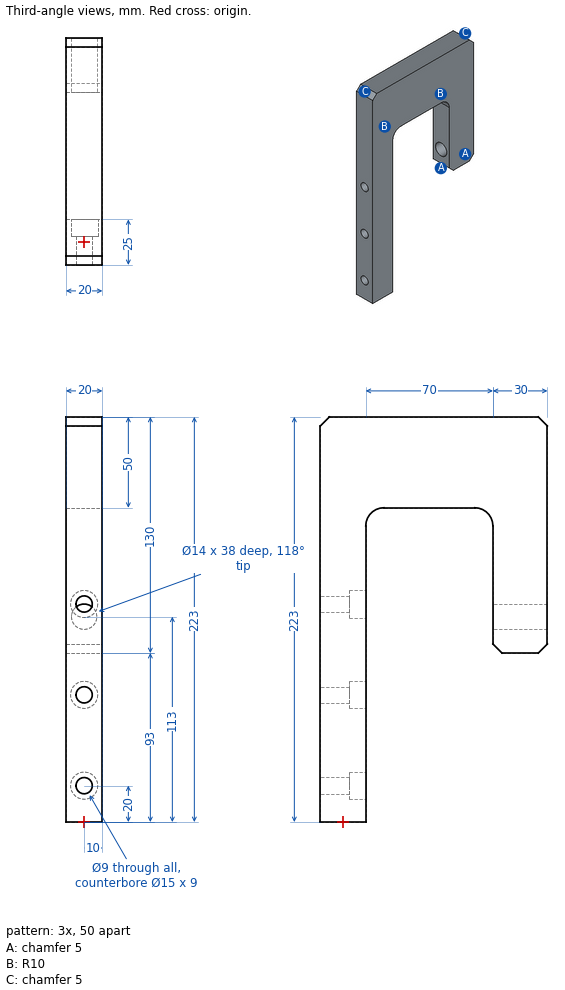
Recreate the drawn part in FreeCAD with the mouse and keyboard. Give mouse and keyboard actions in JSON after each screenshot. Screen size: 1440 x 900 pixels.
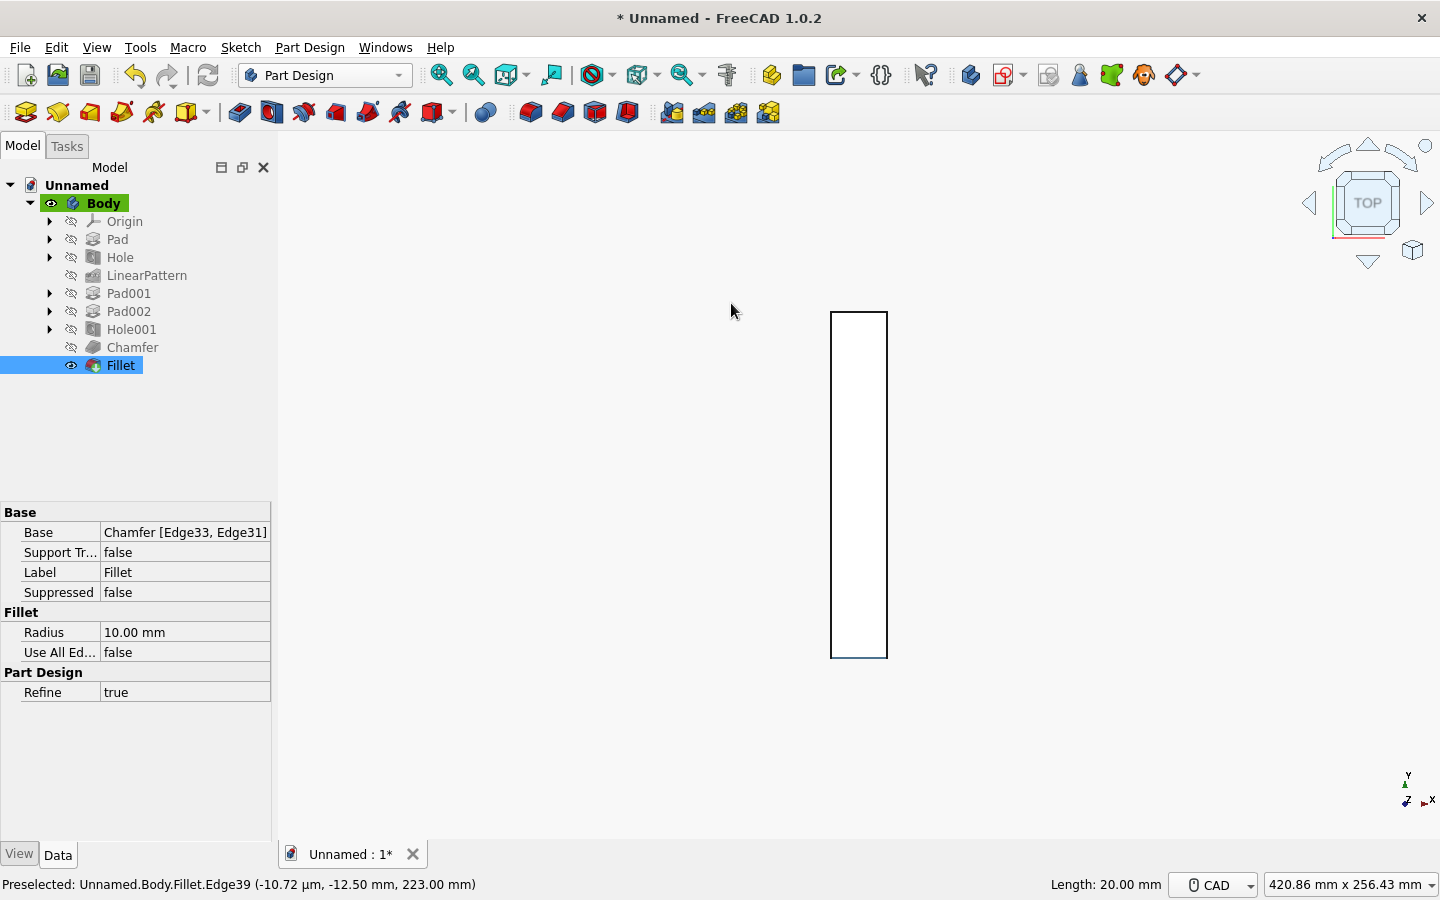
{"action": "left_click", "coordinate": [859, 311], "text": "ctrl"}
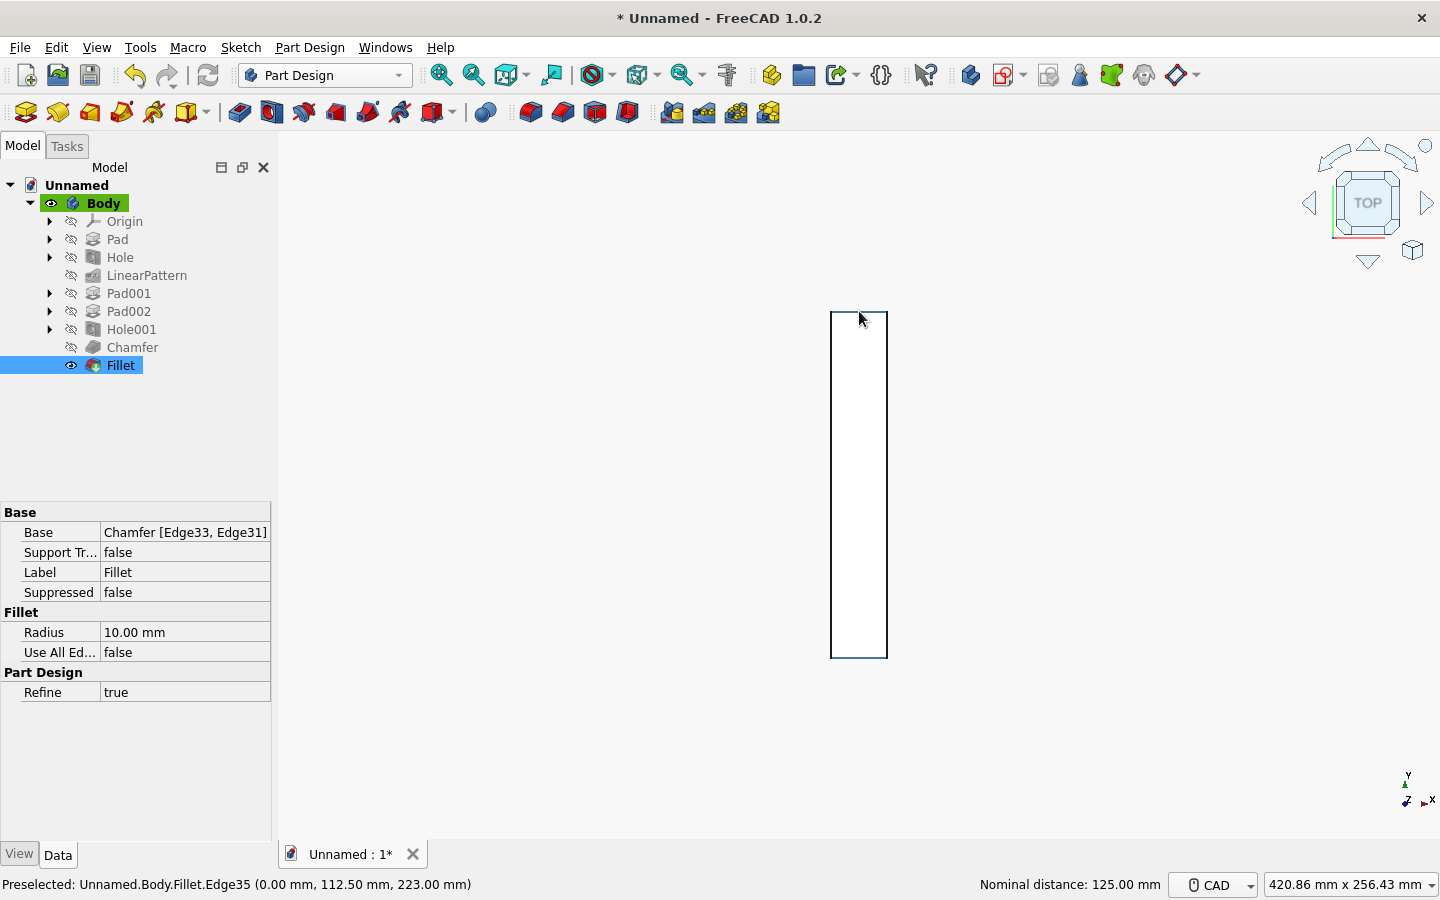
{"action": "left_click", "coordinate": [564, 112]}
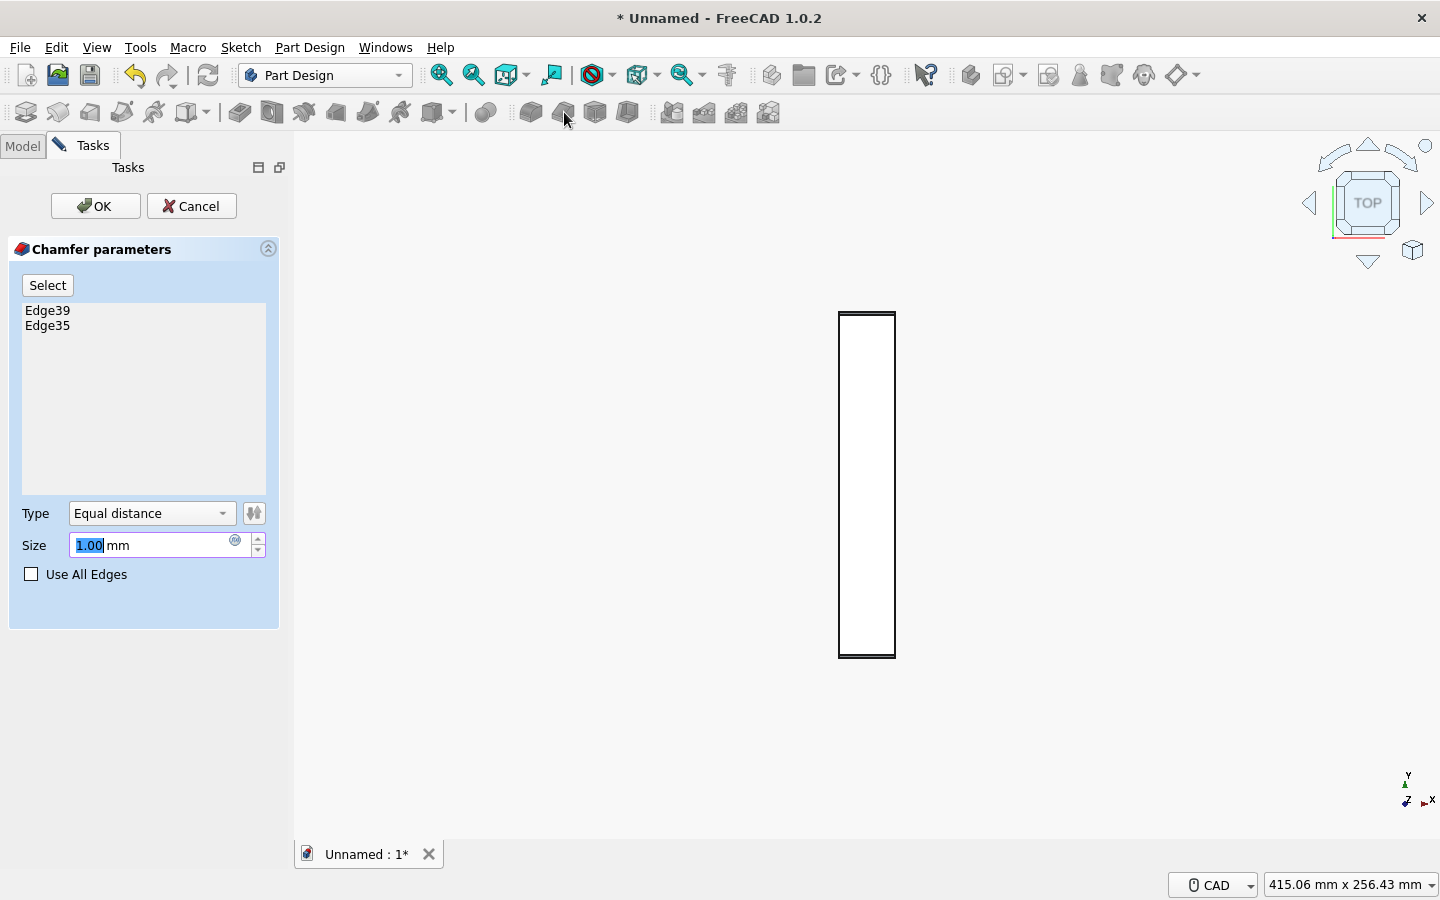
{"action": "type", "text": "5"}
{"action": "key", "text": "Tab"}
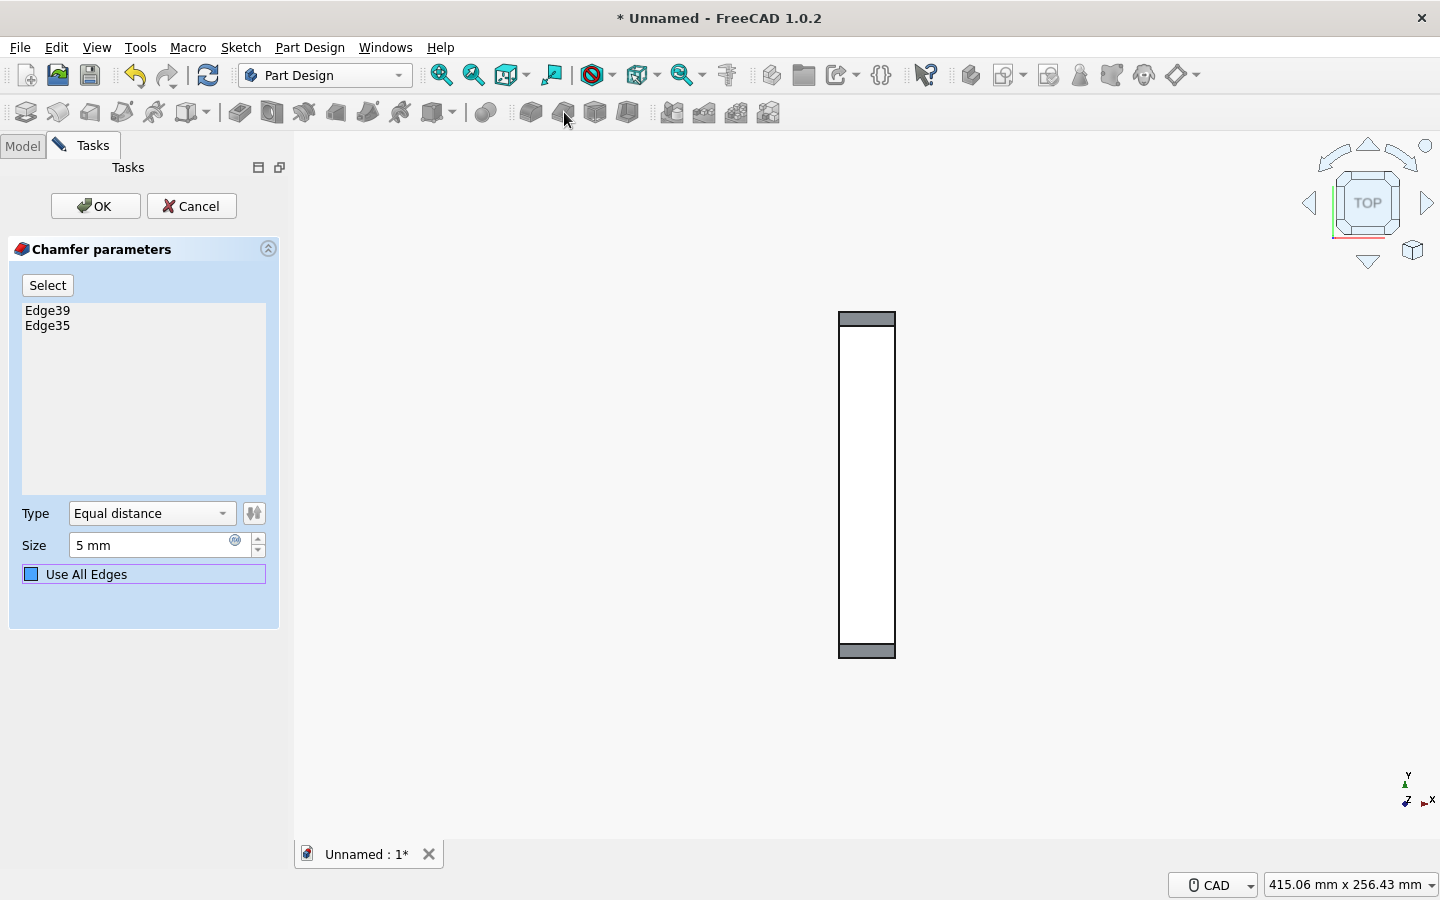
{"action": "left_click", "coordinate": [96, 206]}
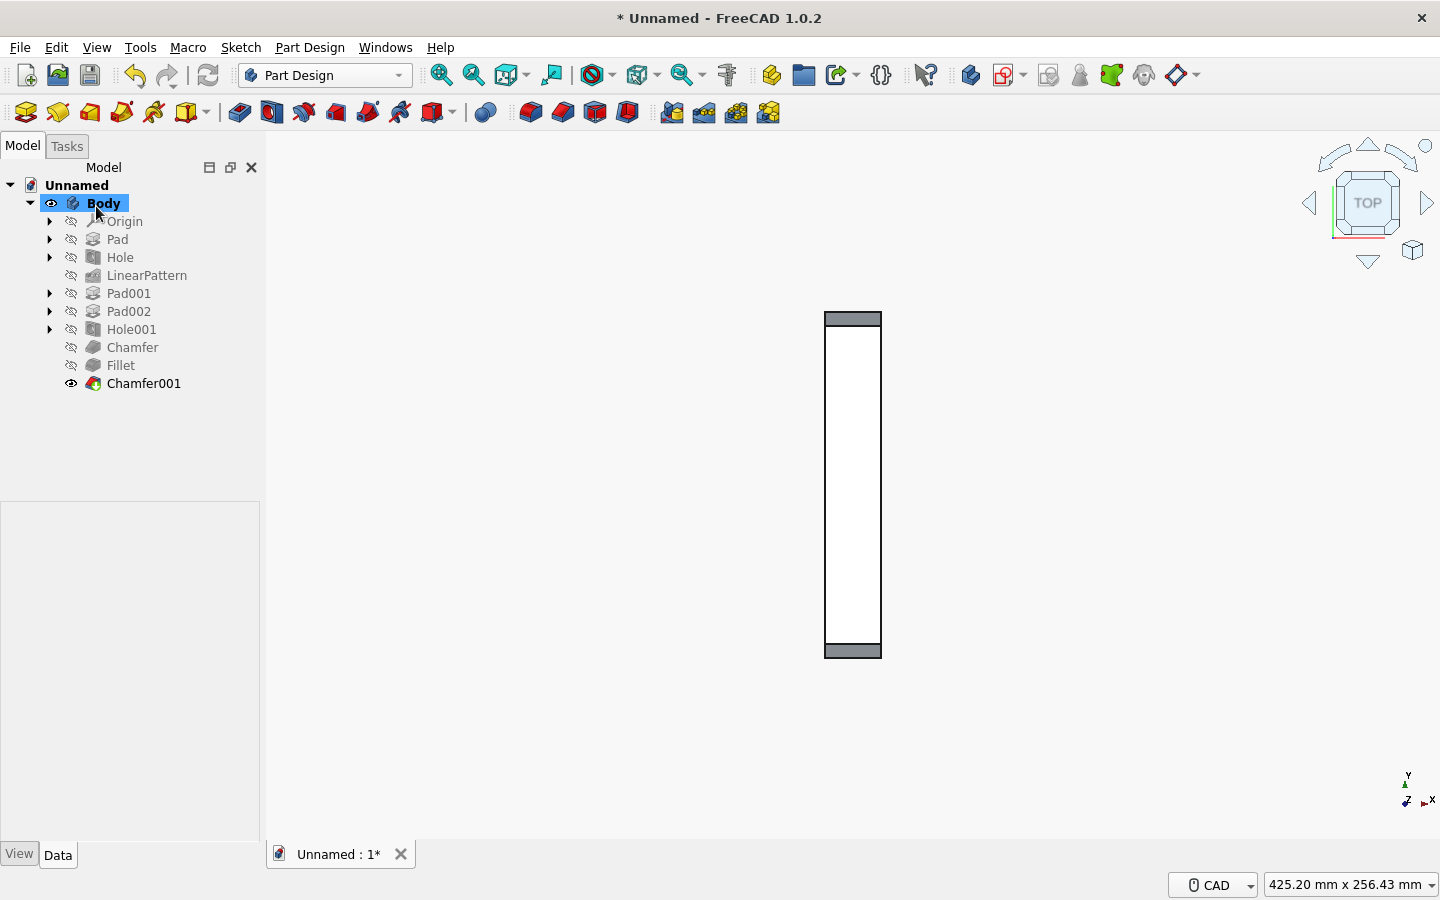
{"action": "key", "text": "0"}